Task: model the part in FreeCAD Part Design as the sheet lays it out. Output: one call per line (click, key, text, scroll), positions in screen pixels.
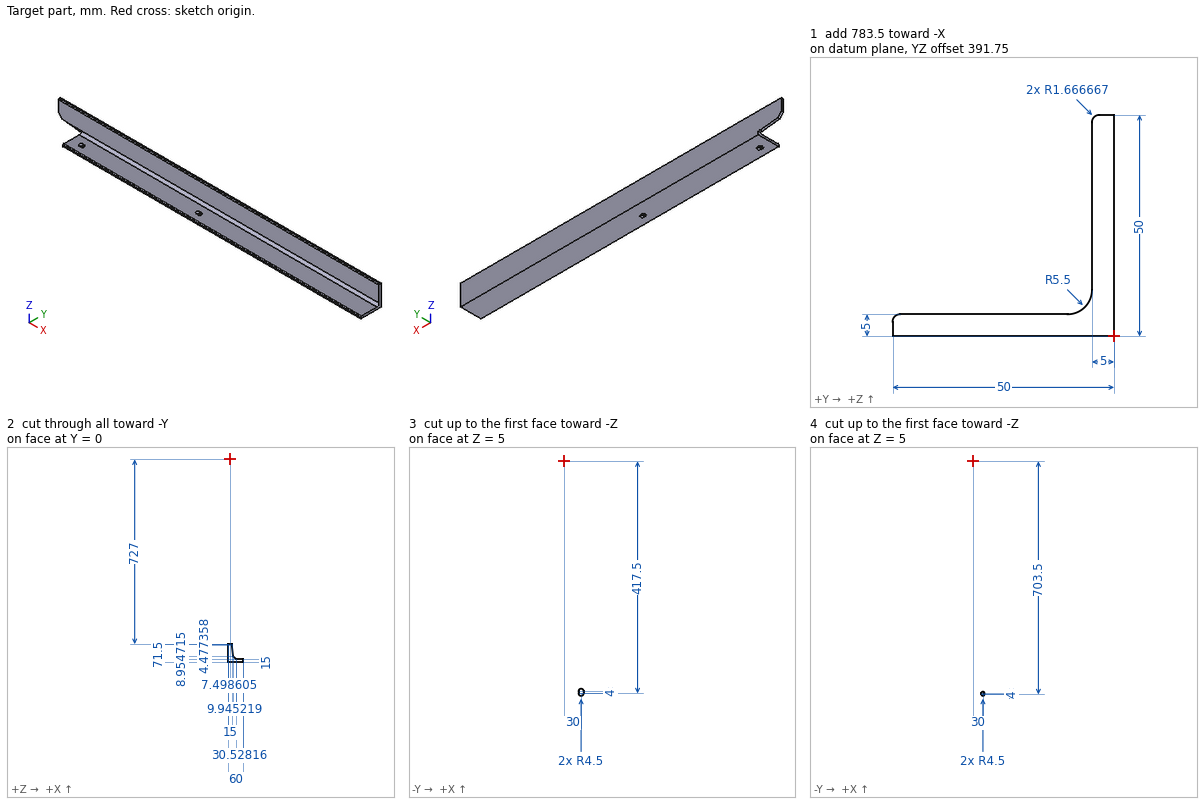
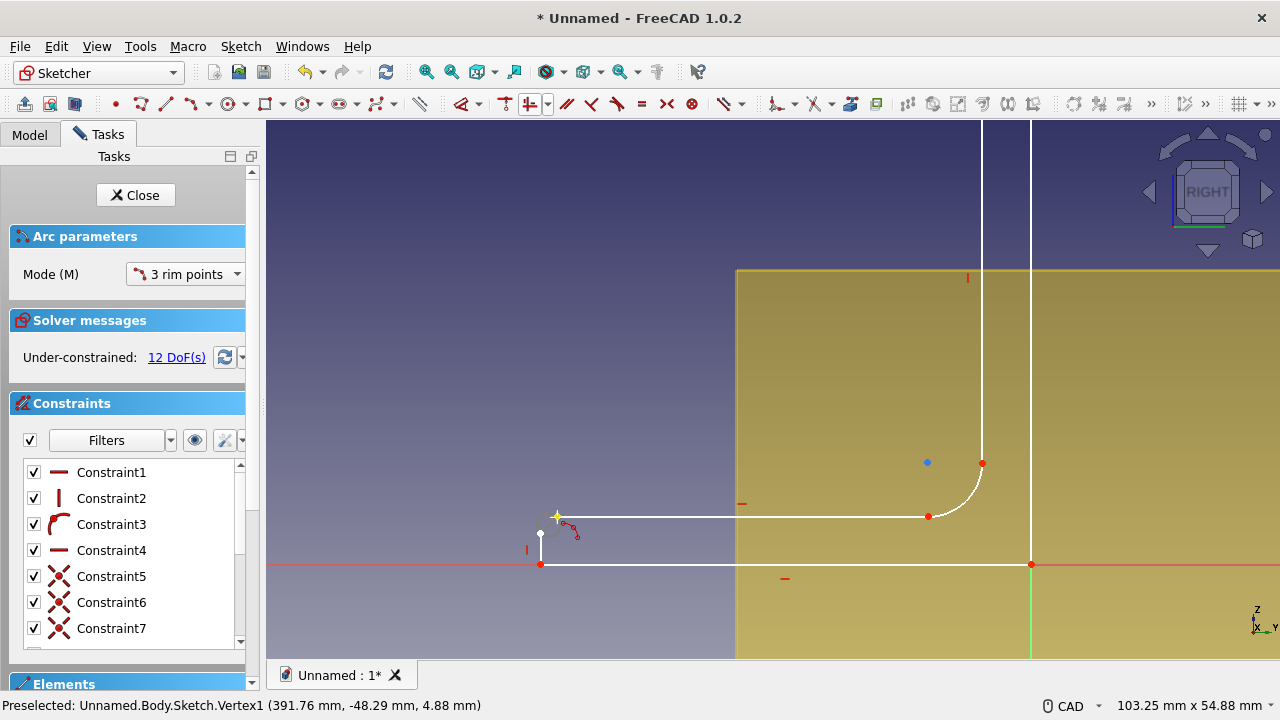
scroll(545, 521, up, 6)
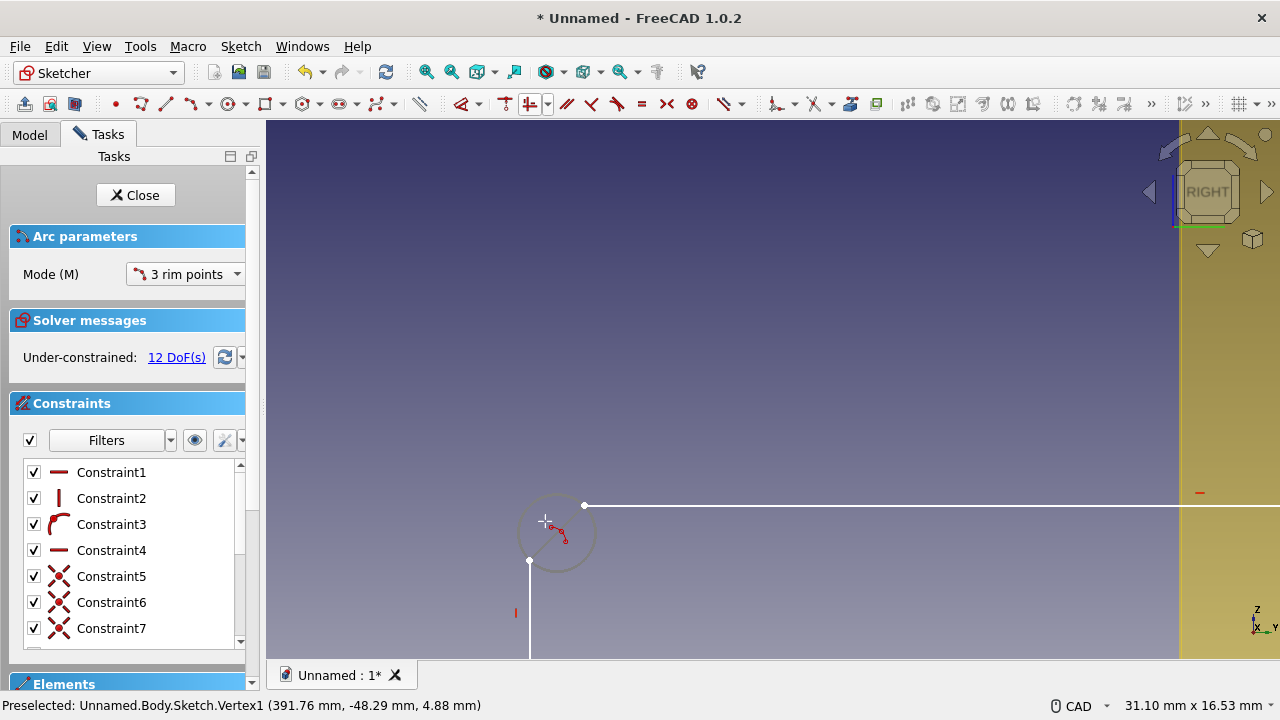
click(544, 518)
key(Escape)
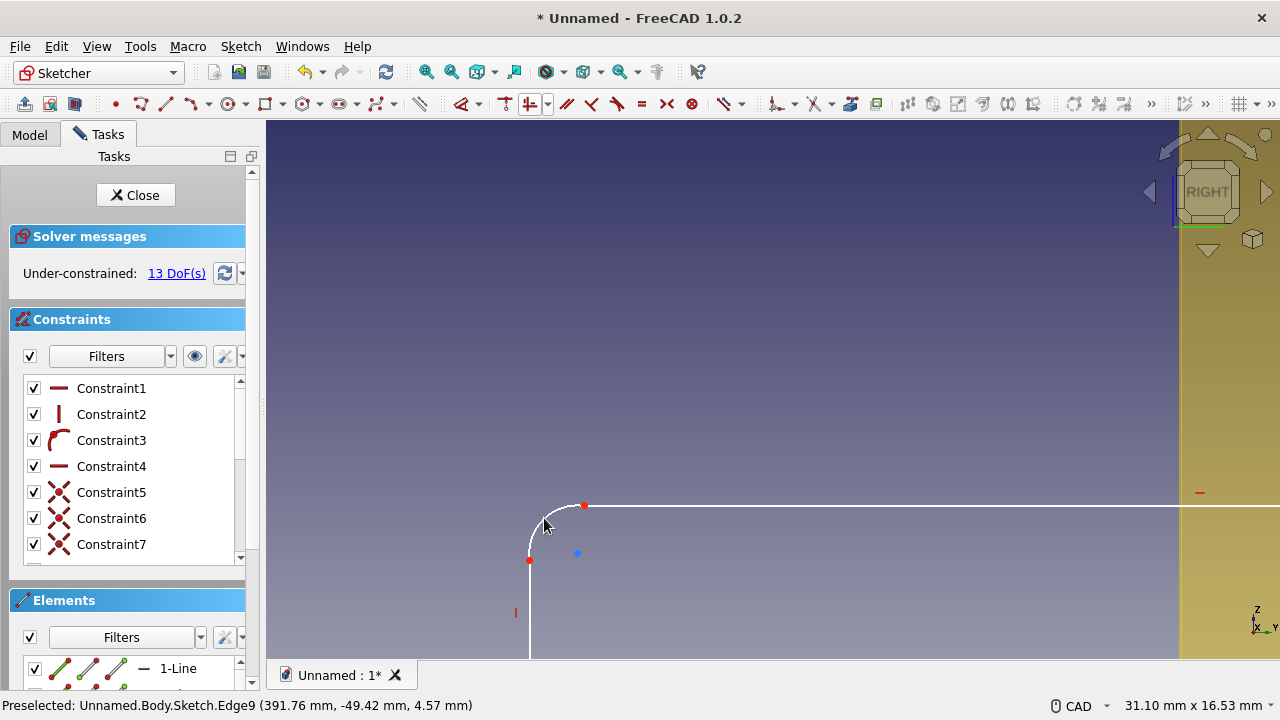
scroll(543, 526, down, 8)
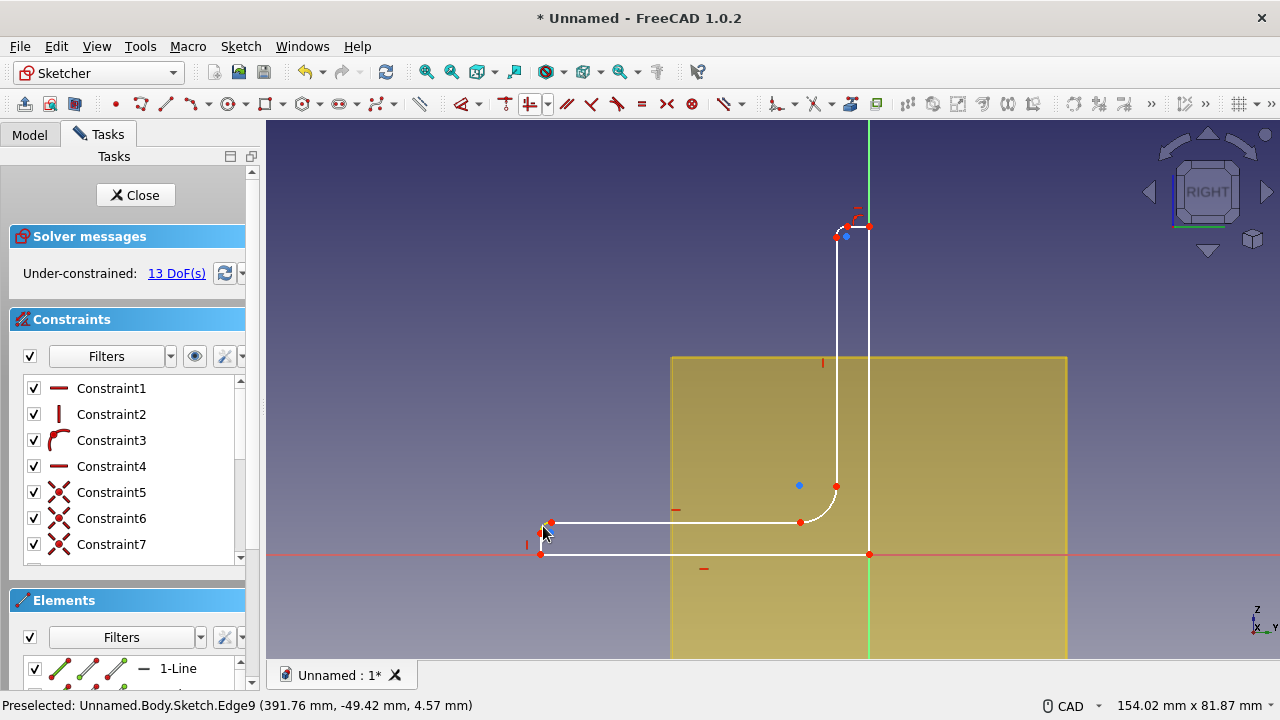
click(626, 523)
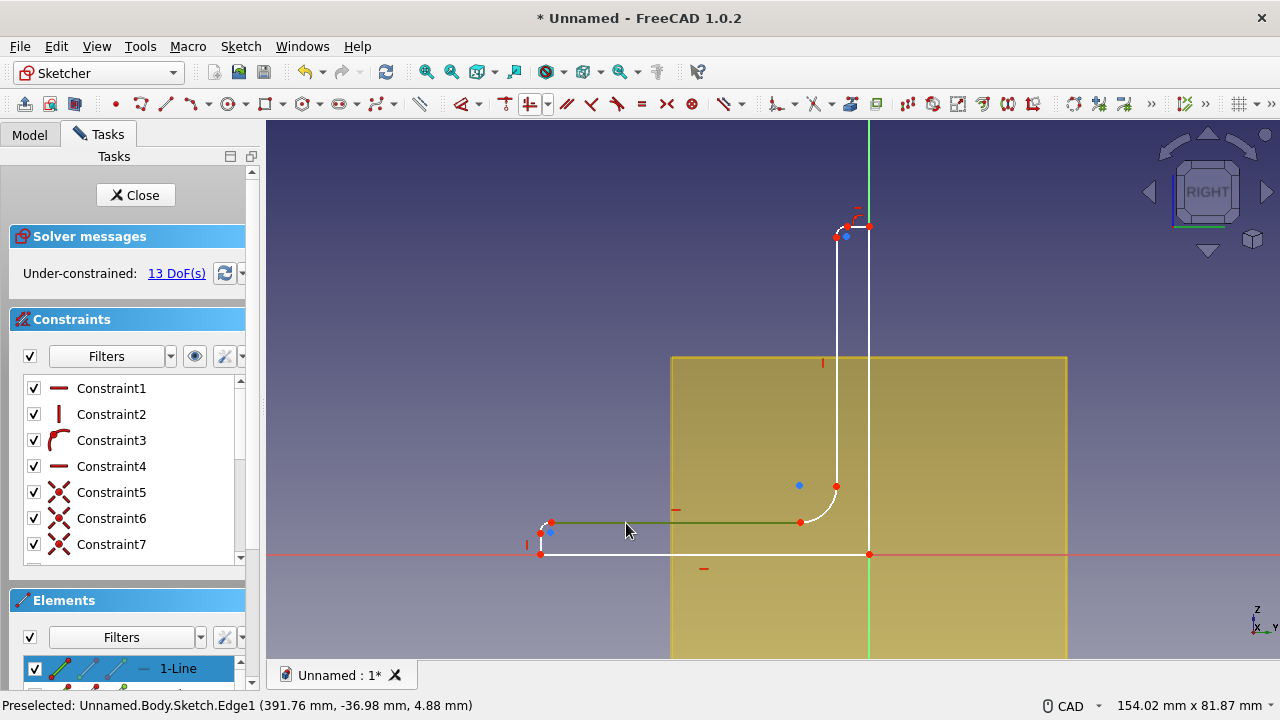
click(817, 518)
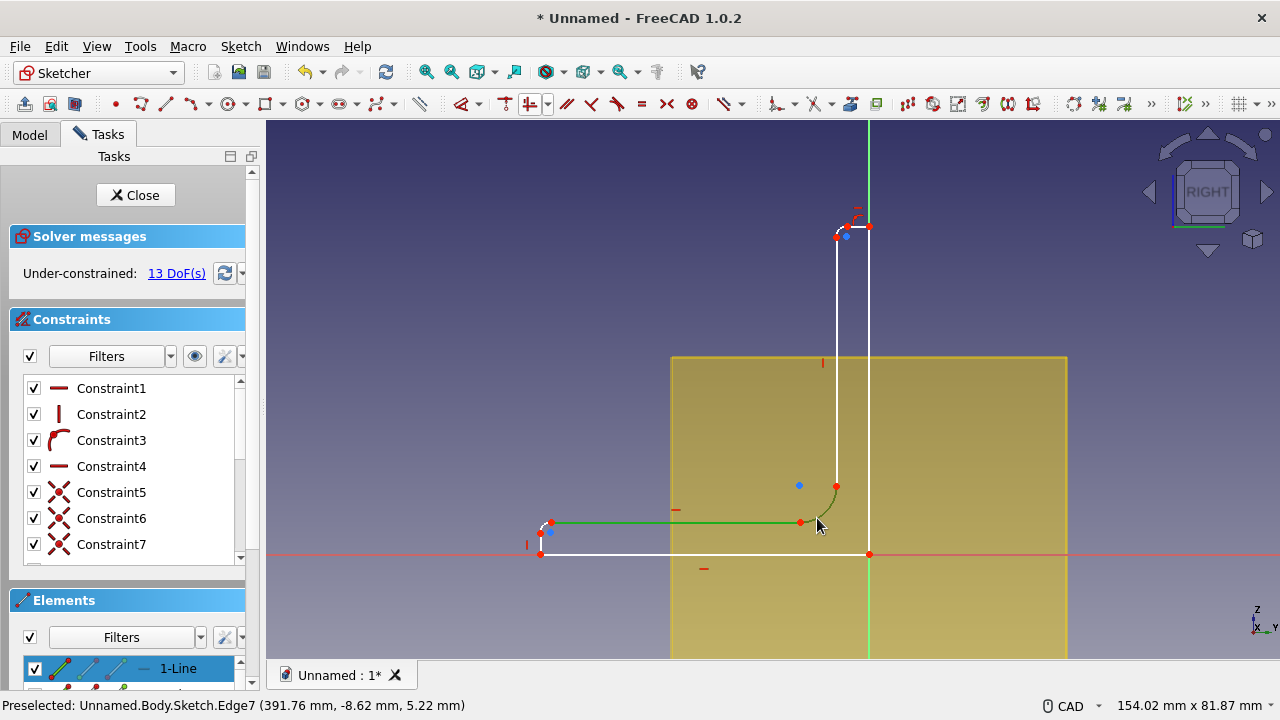
click(617, 104)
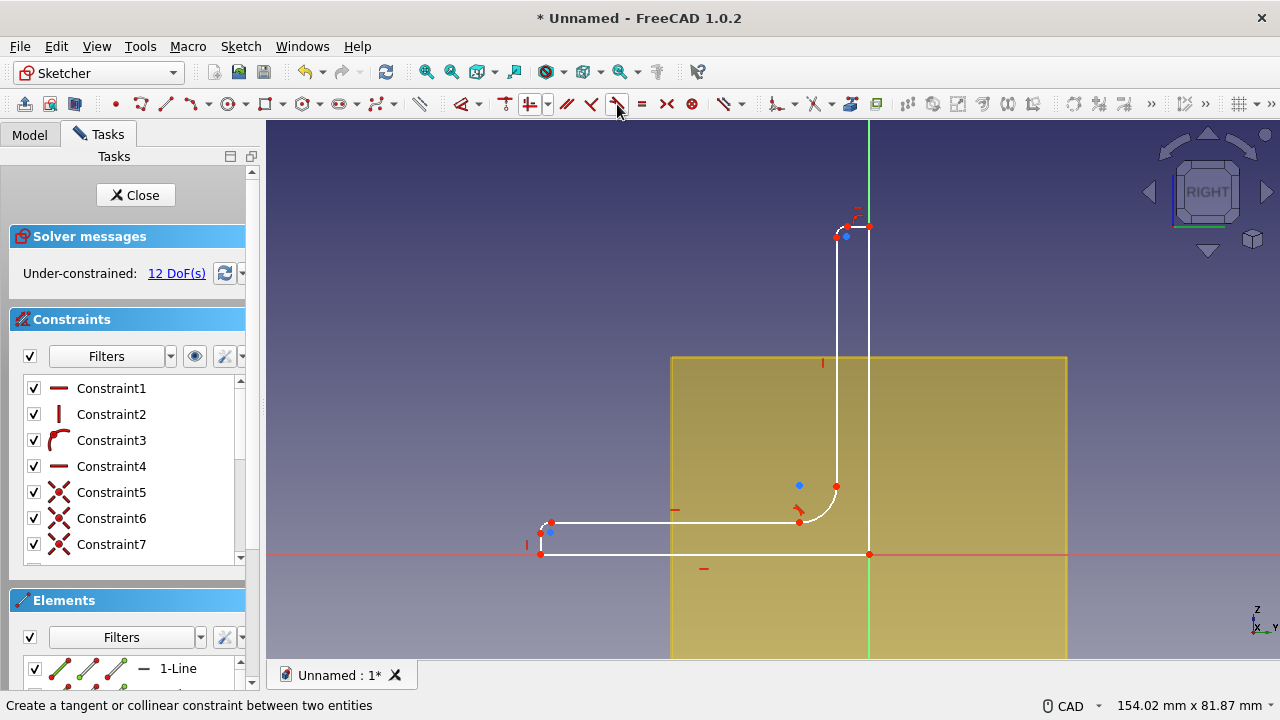
click(626, 523)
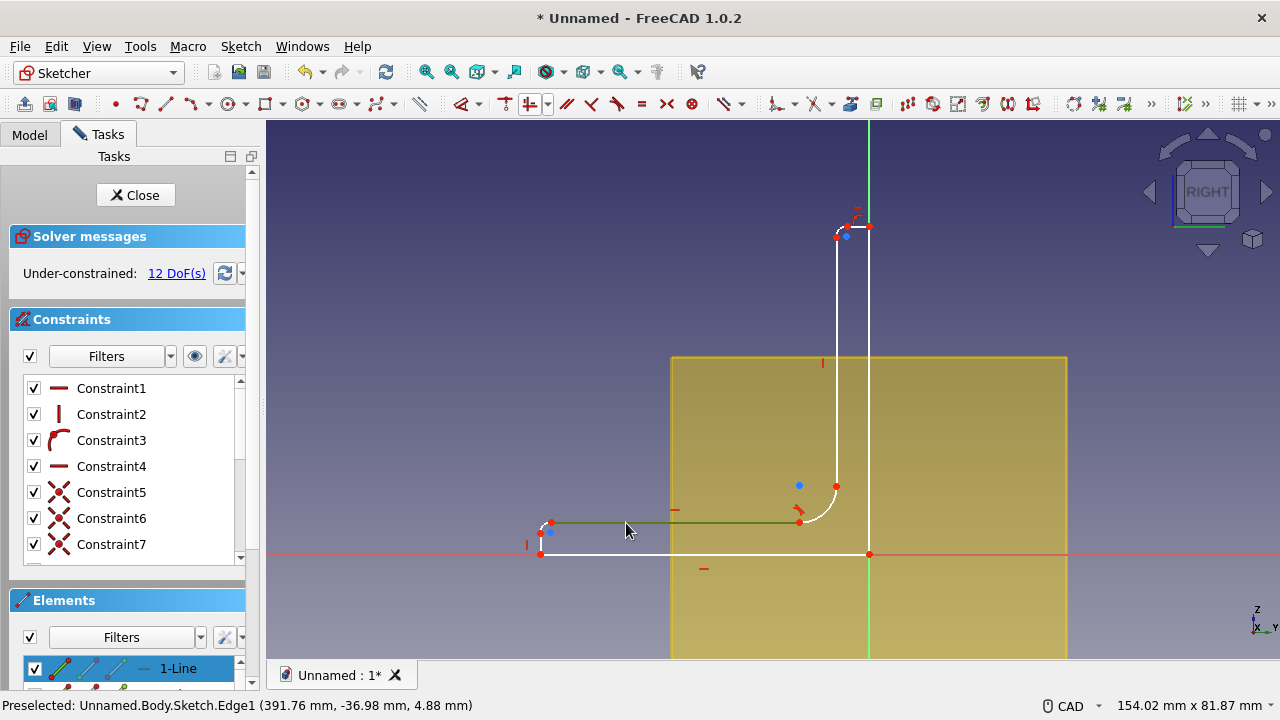
scroll(543, 525, up, 3)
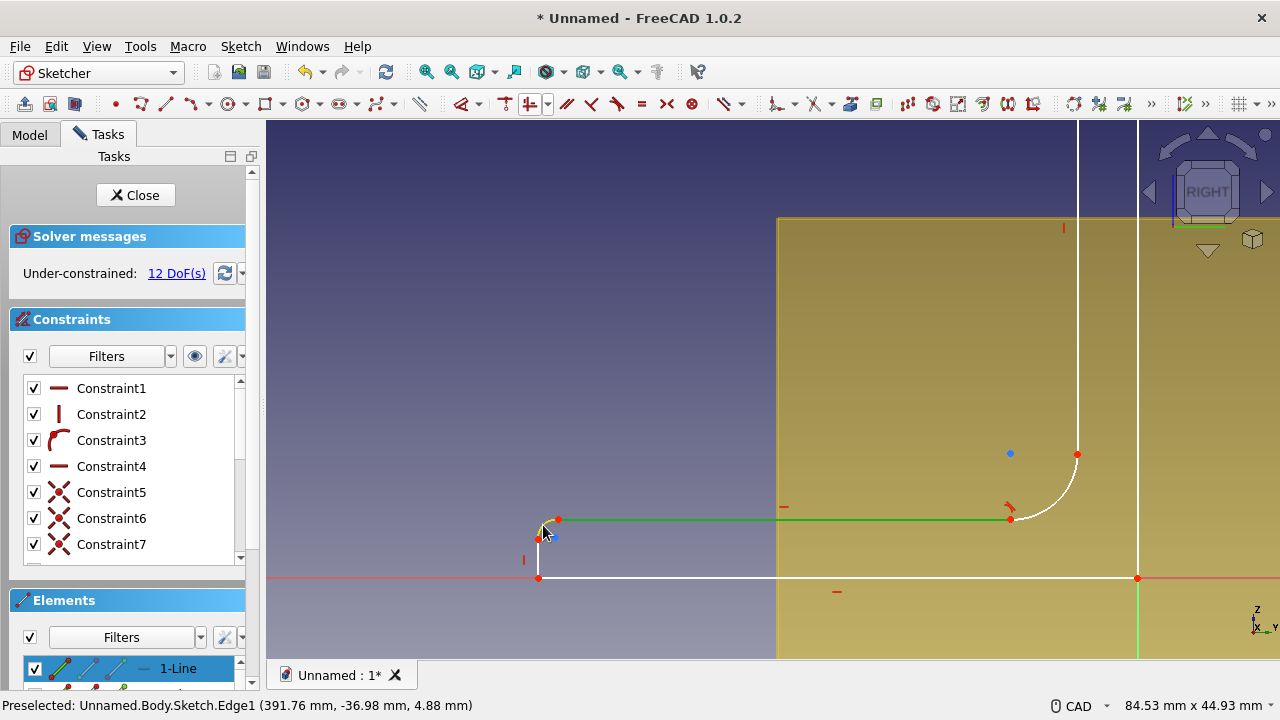
click(543, 525)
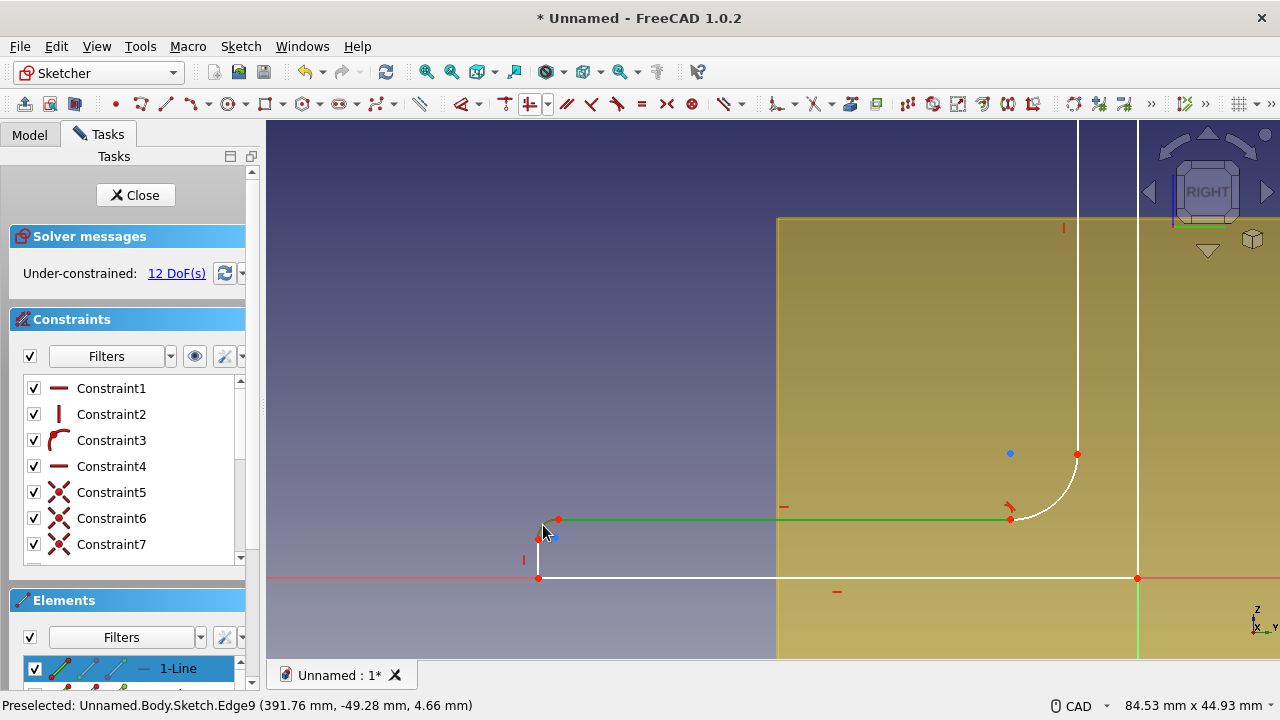
click(617, 104)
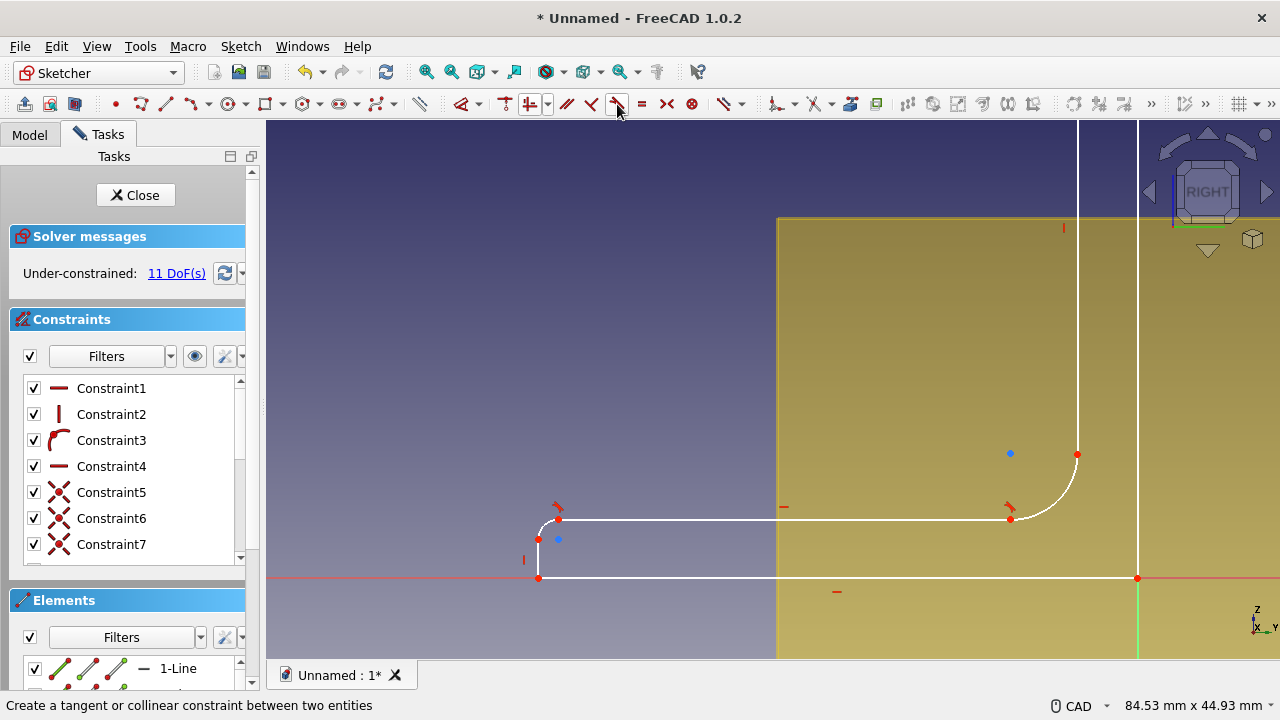
click(1078, 318)